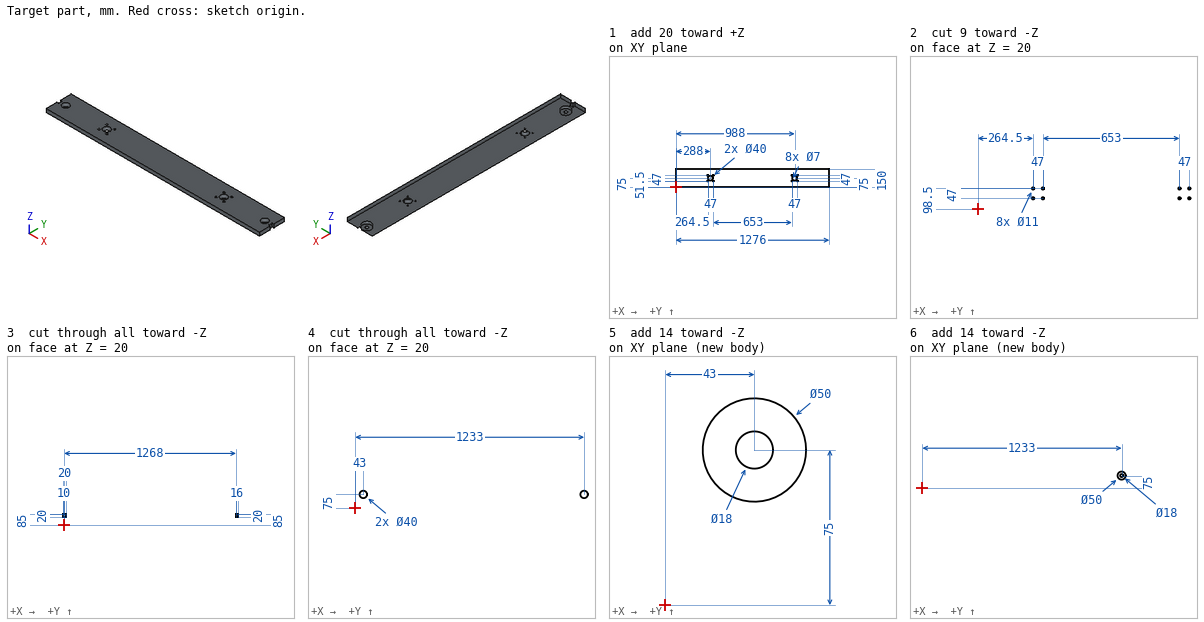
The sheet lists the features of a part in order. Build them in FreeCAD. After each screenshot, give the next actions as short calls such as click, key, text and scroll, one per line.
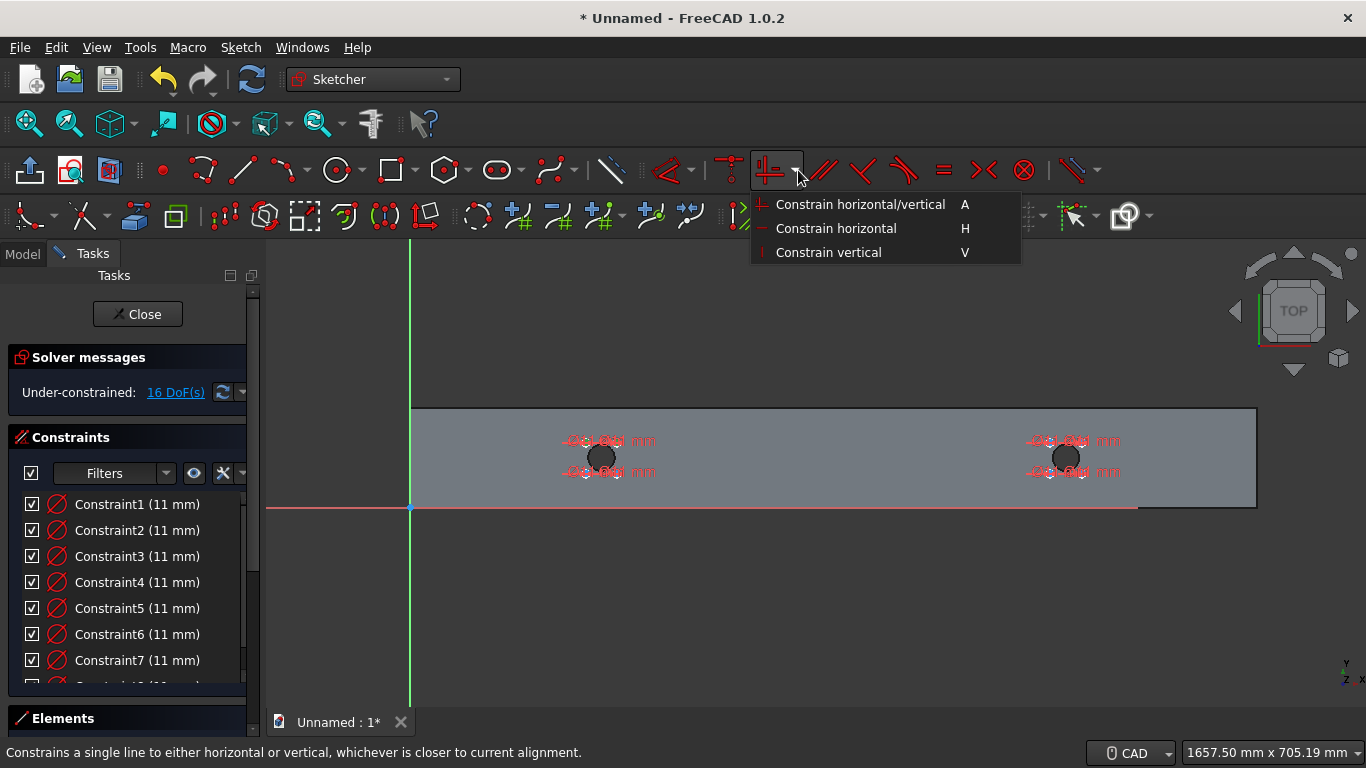
click(886, 228)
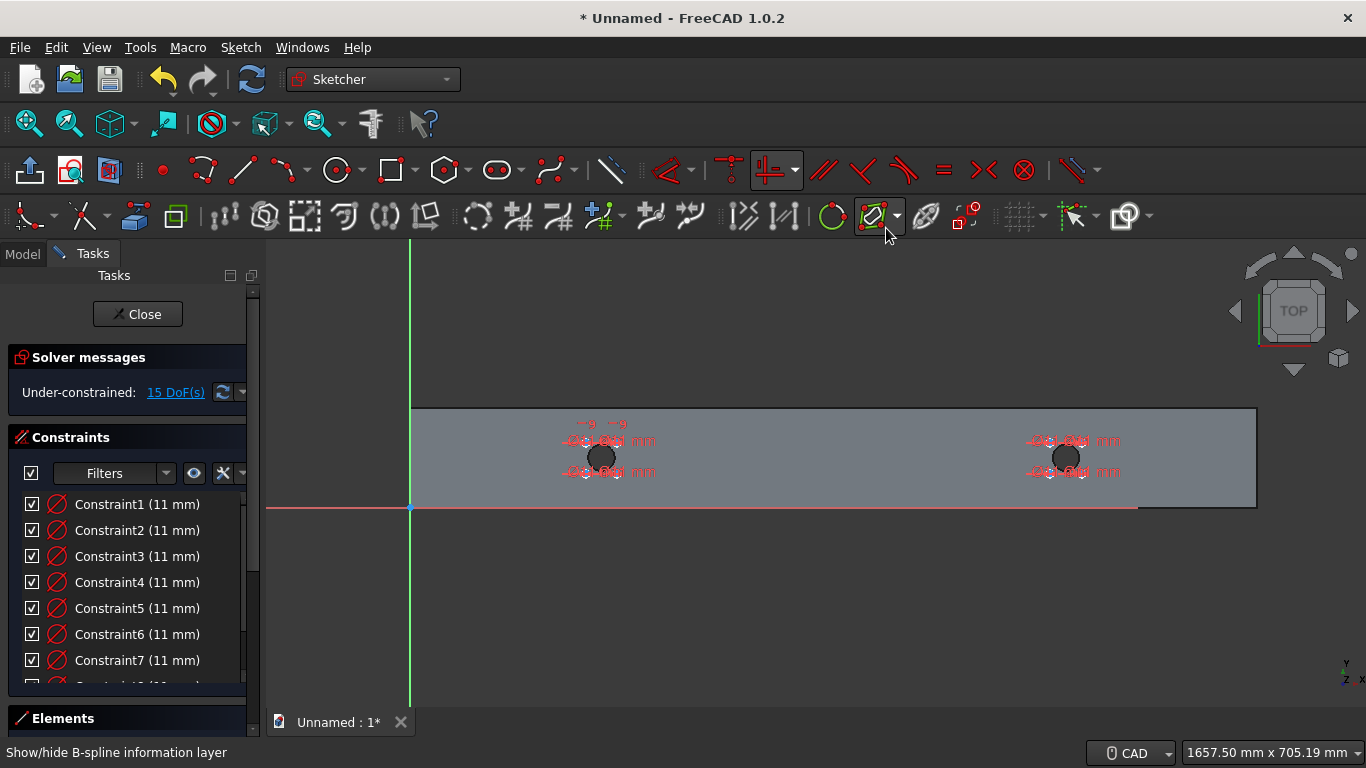
click(617, 443)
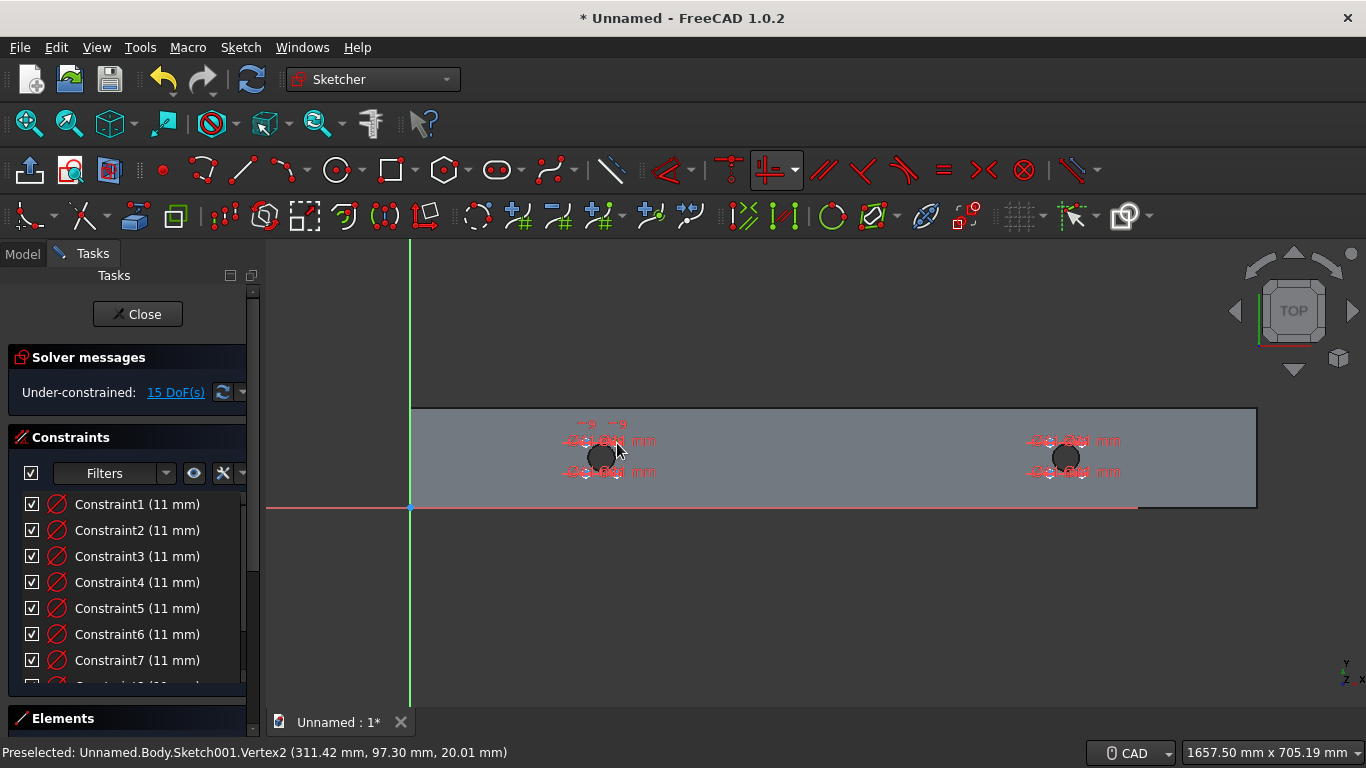
click(617, 474)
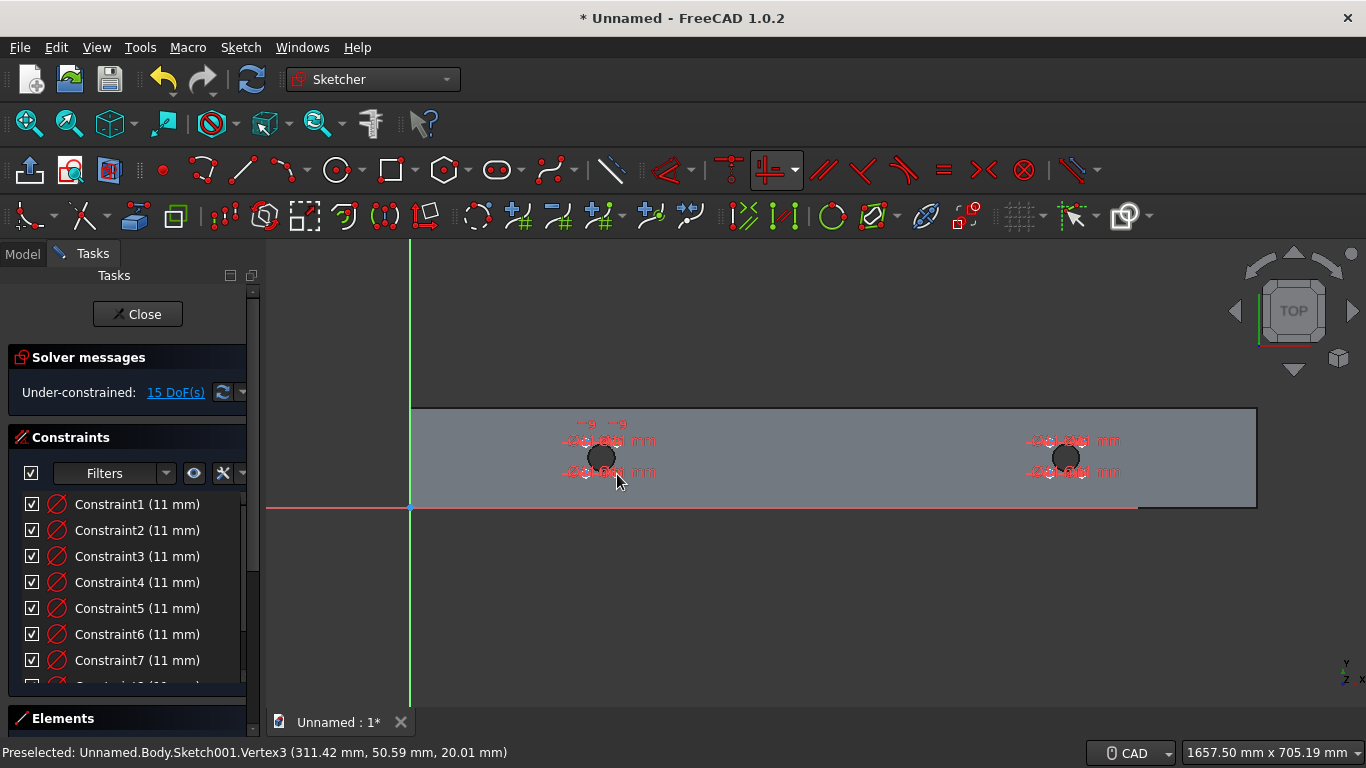
click(798, 170)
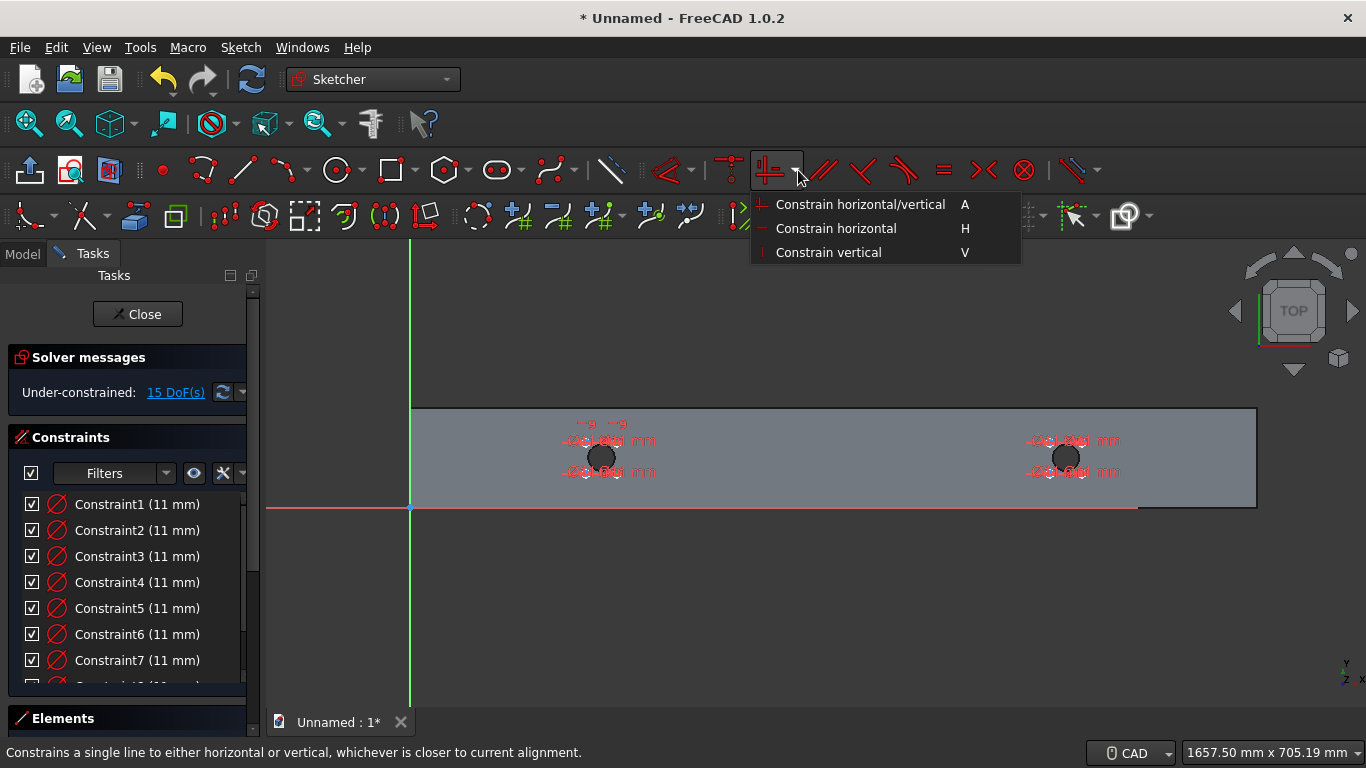
click(886, 252)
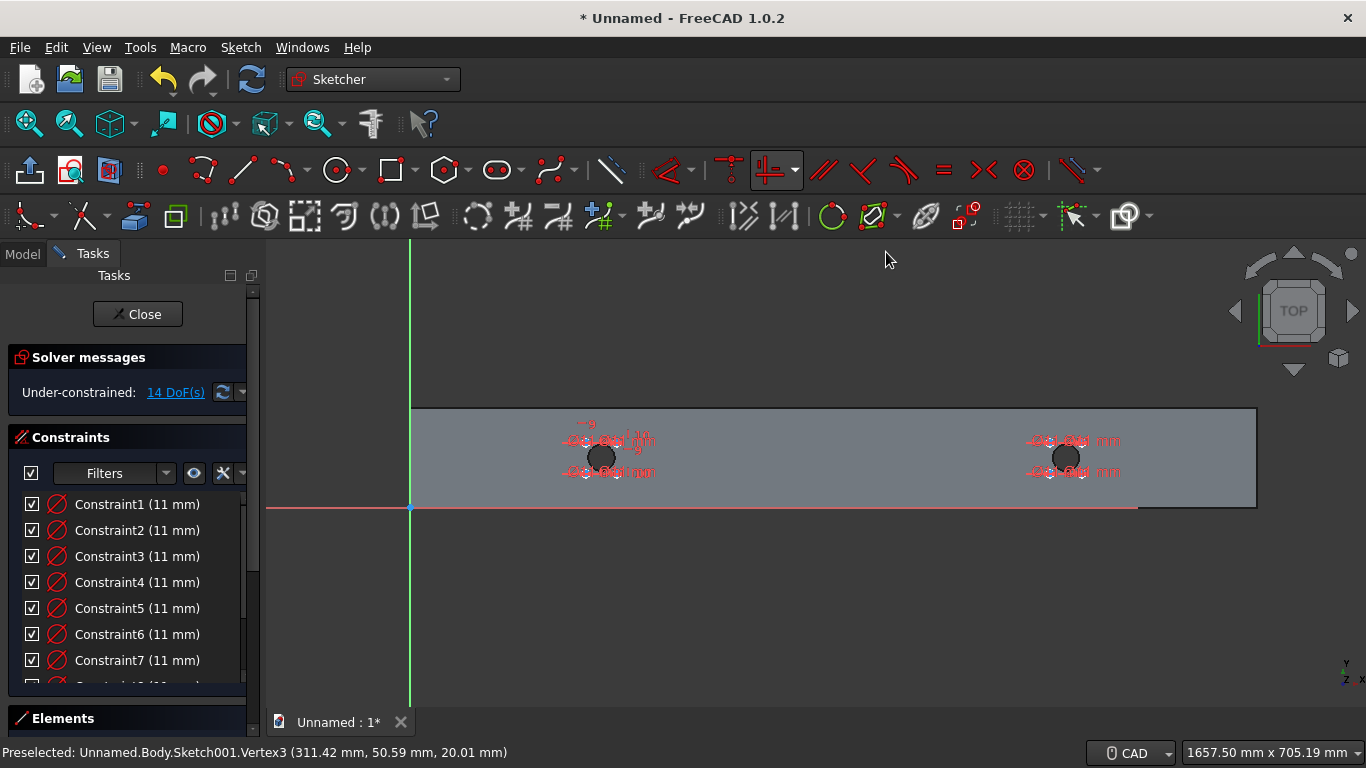
click(586, 443)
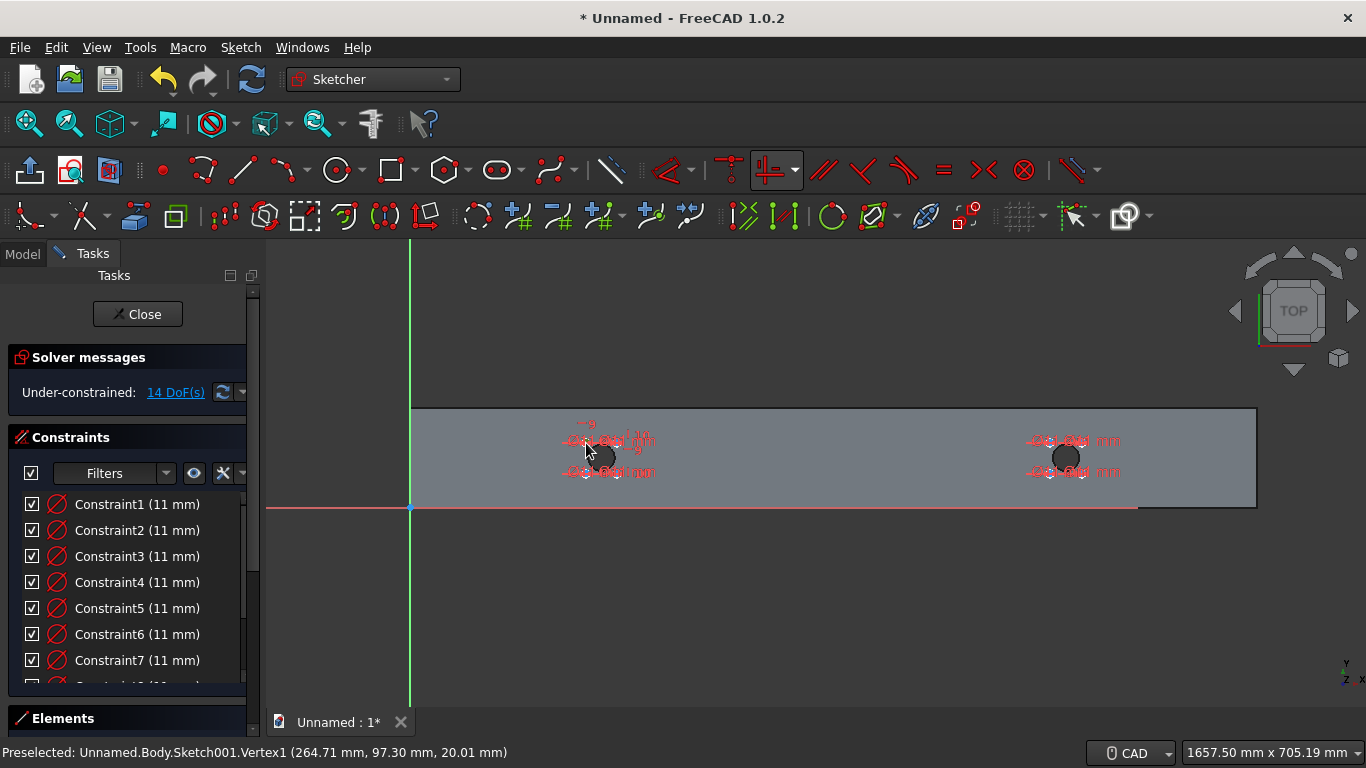
click(586, 474)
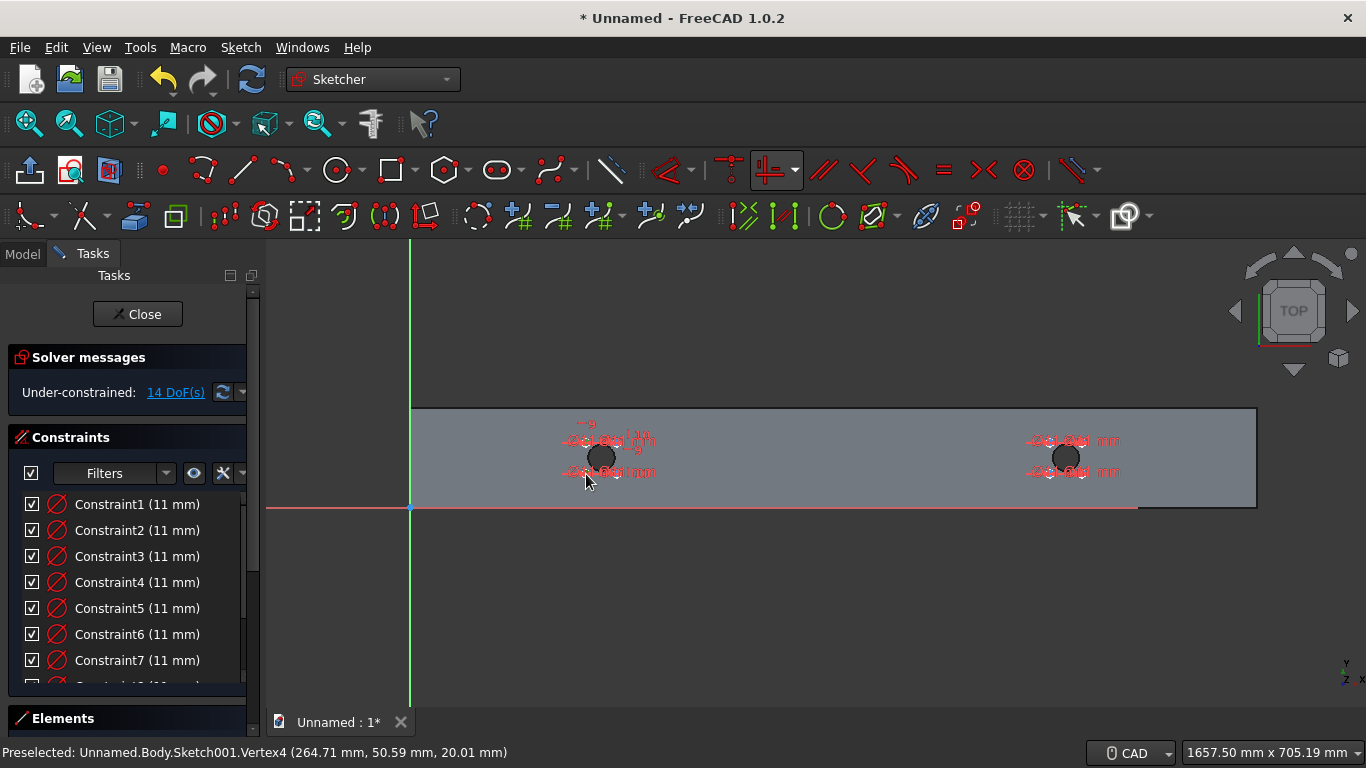
click(798, 170)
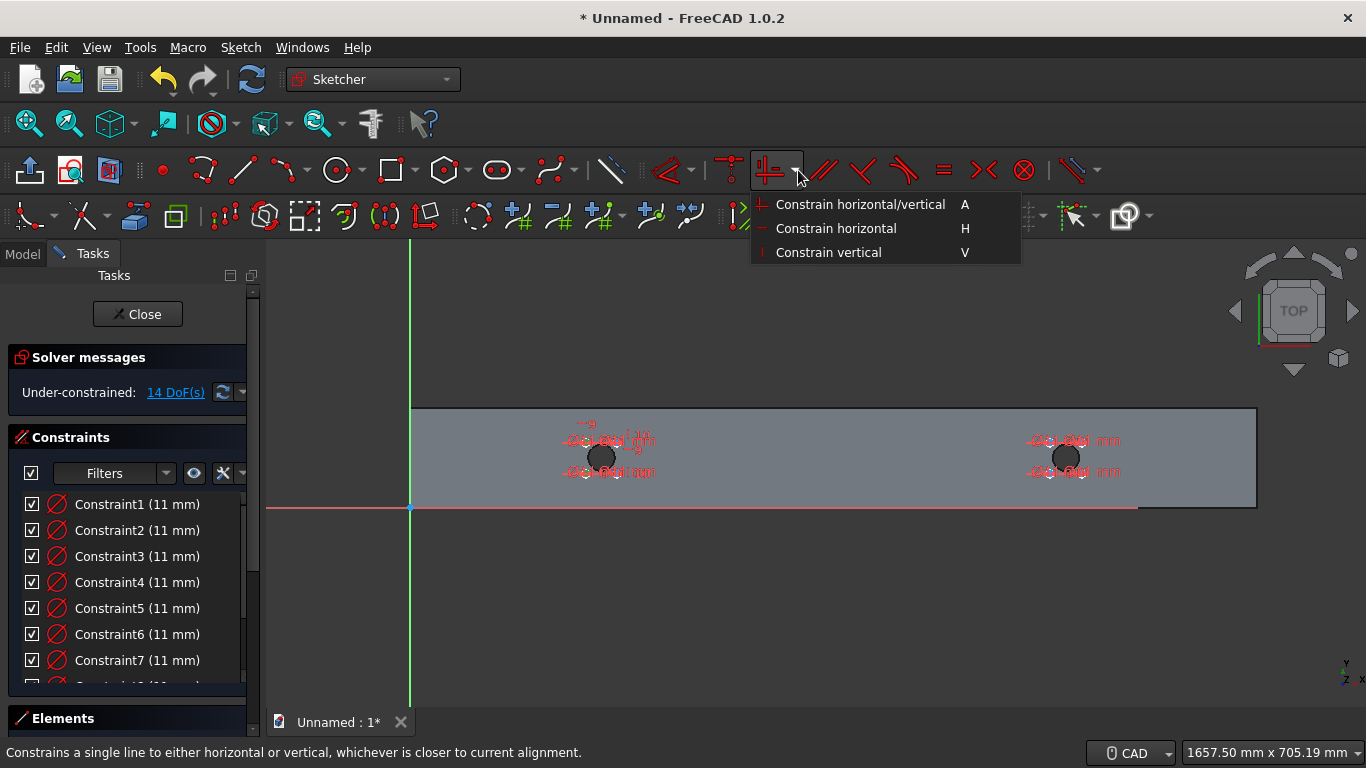
click(886, 252)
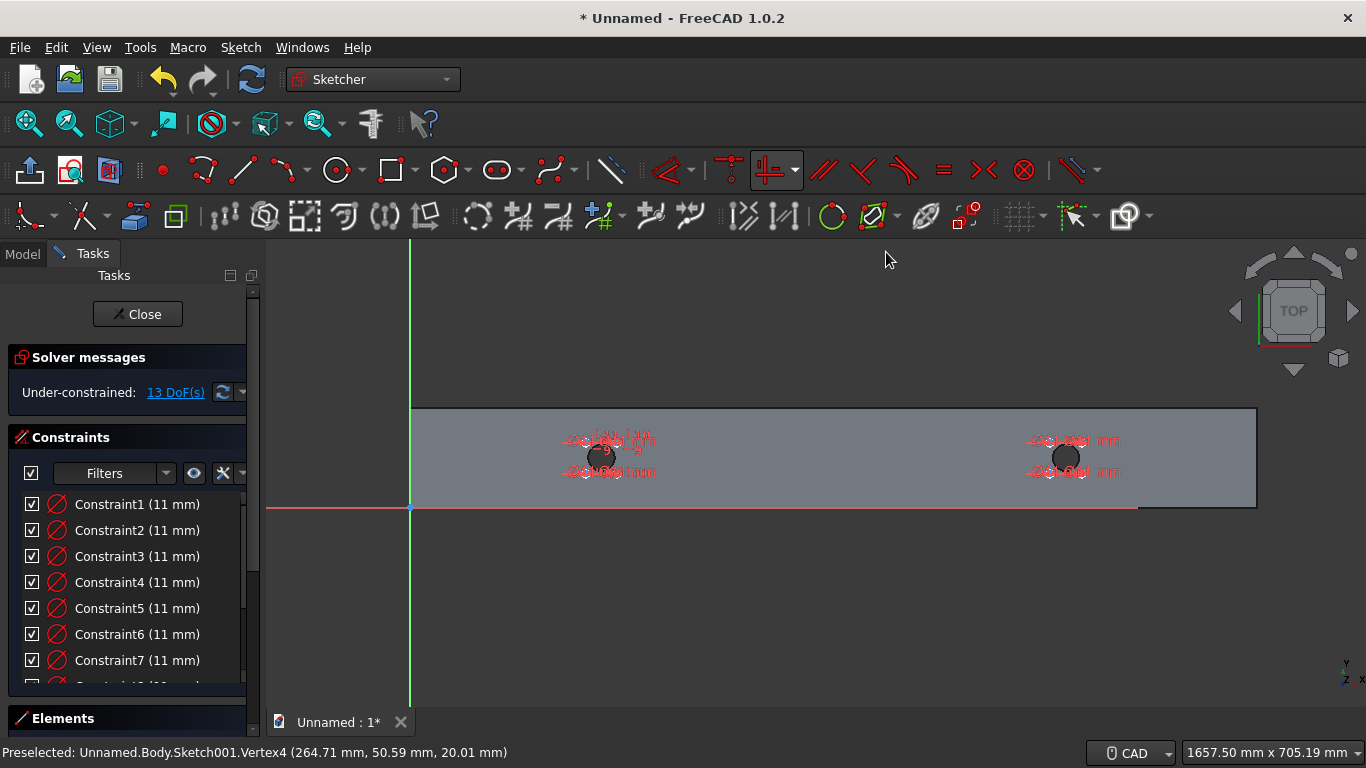
click(619, 476)